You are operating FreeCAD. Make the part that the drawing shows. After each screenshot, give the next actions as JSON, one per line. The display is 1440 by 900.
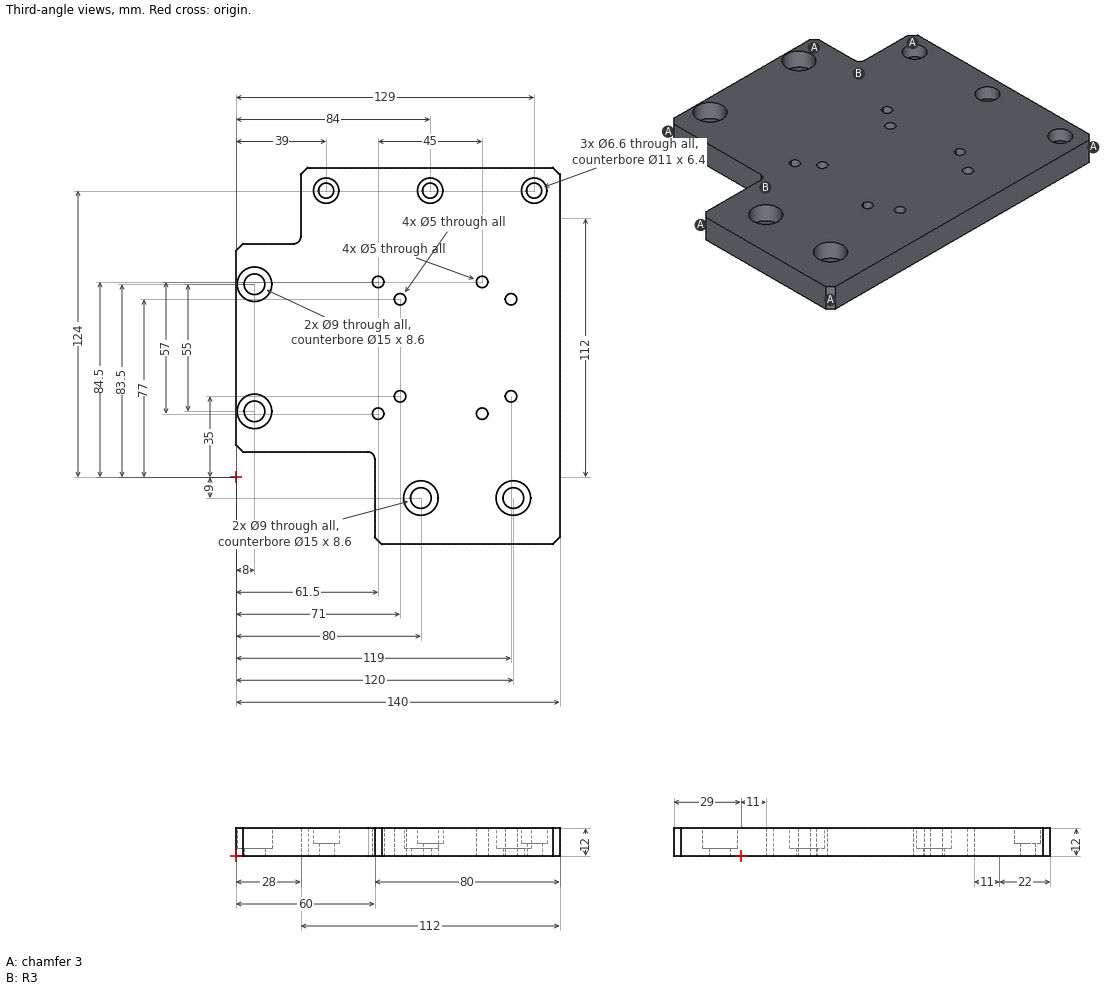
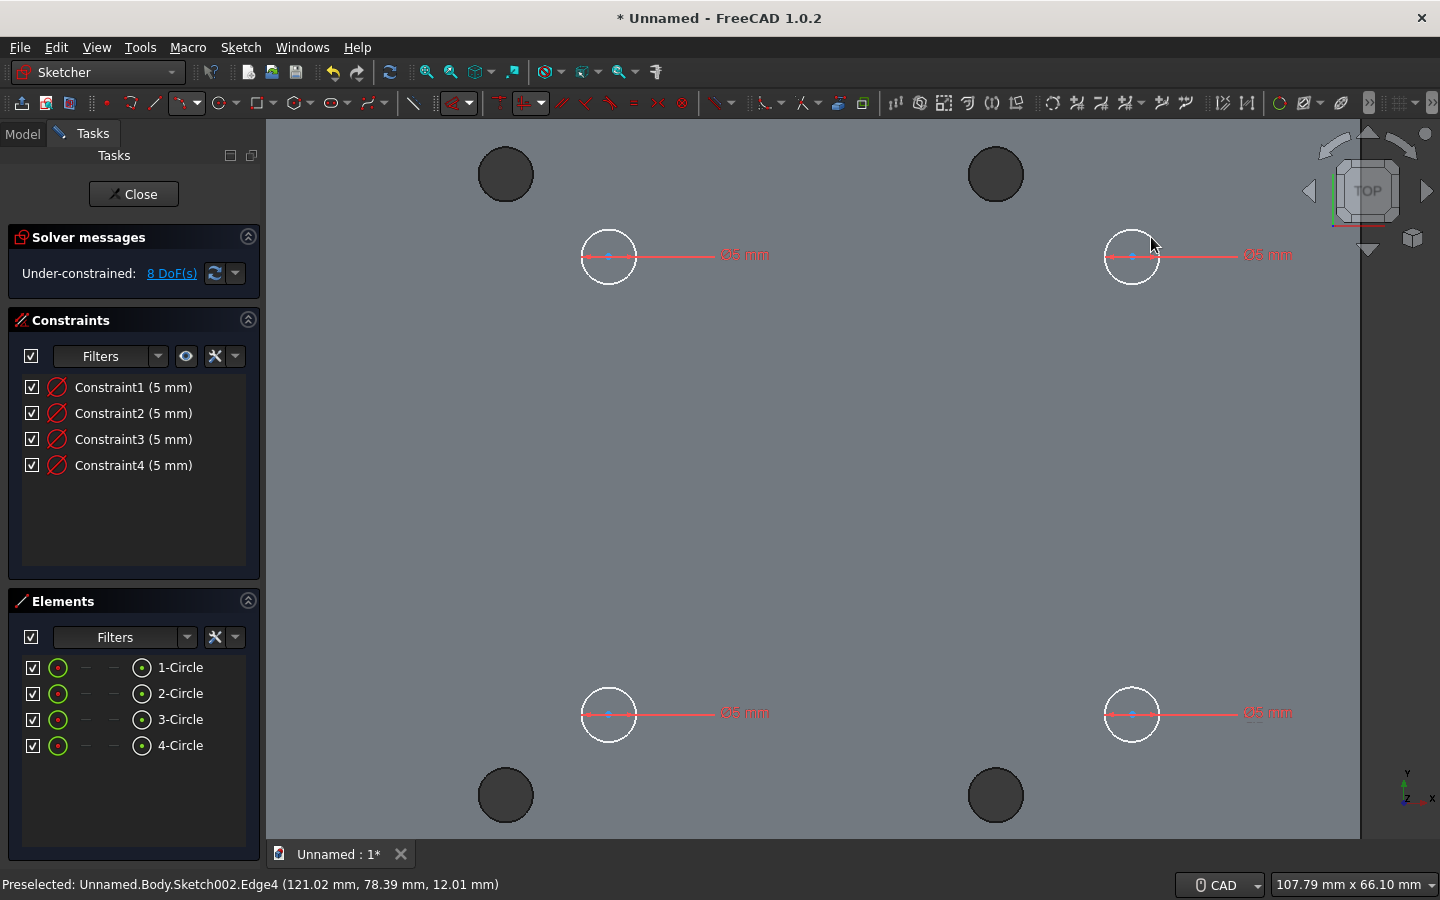
{"action": "left_click", "coordinate": [609, 257]}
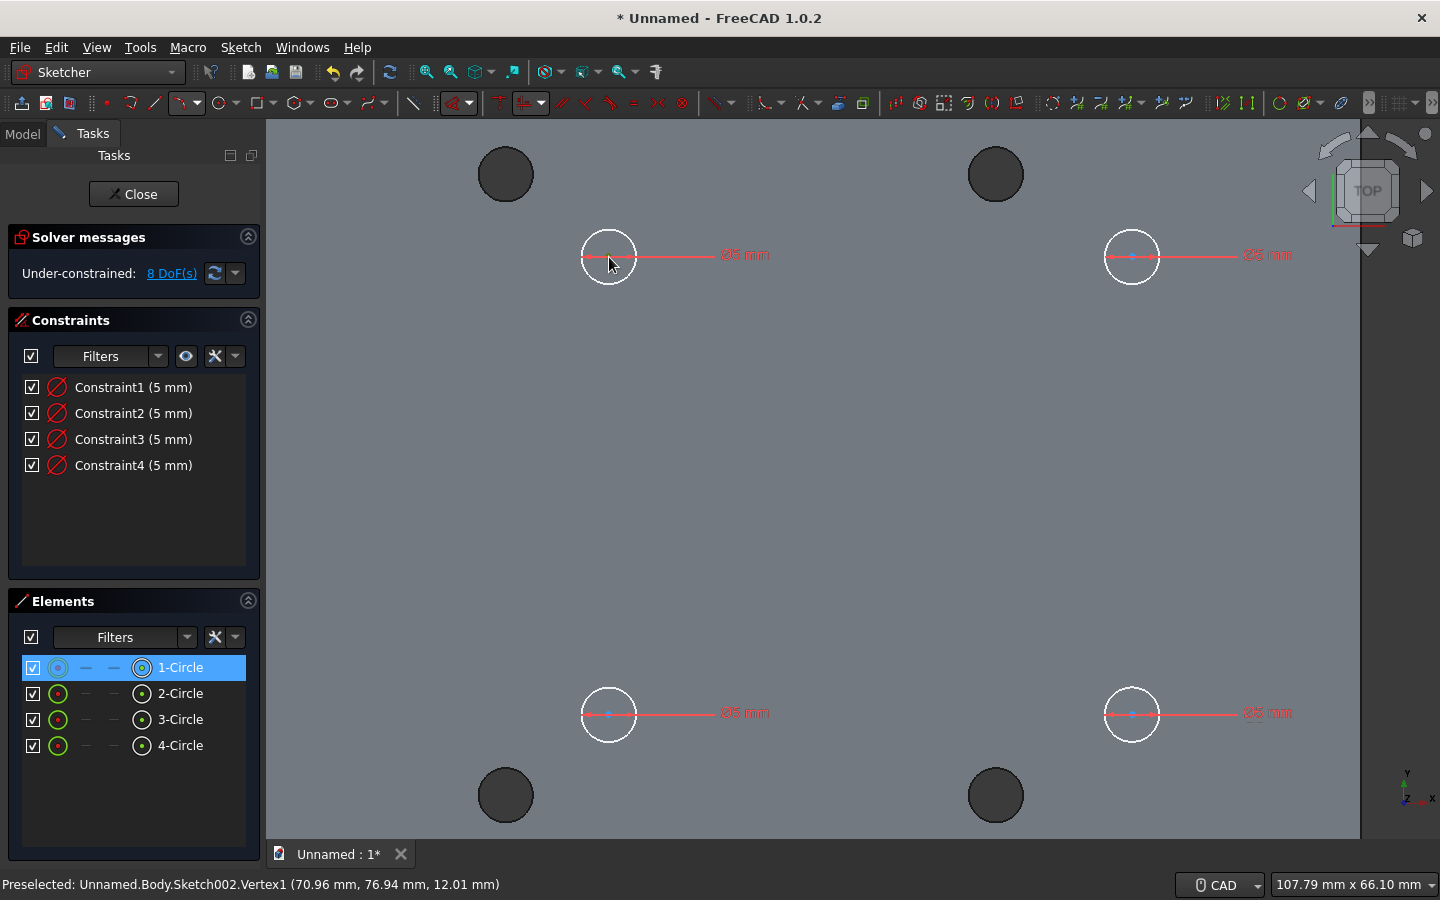
{"action": "key", "text": "l"}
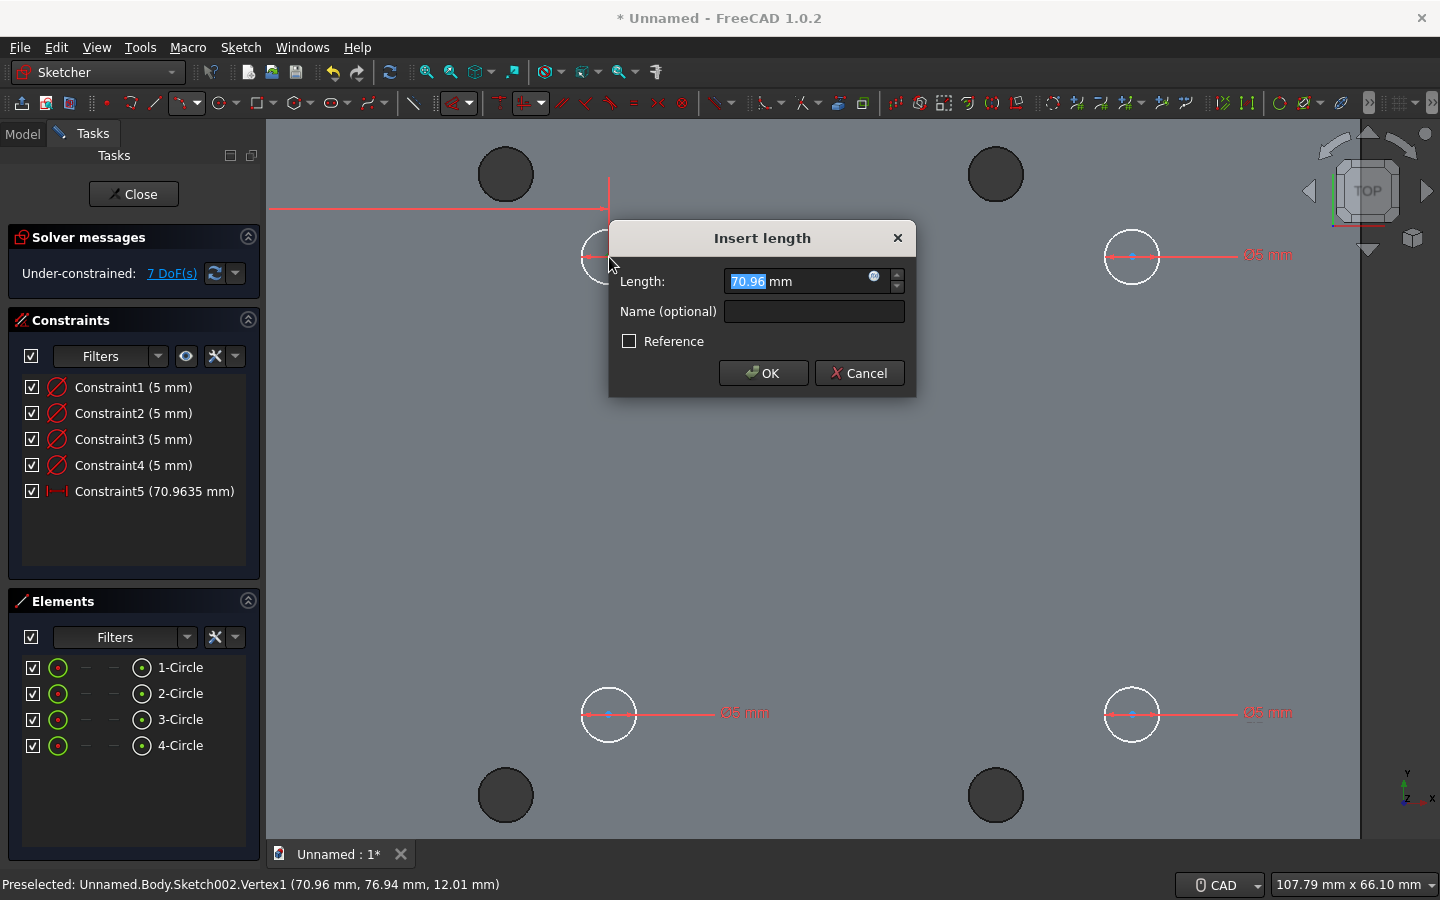
{"action": "type", "text": "71"}
{"action": "key", "text": "Return"}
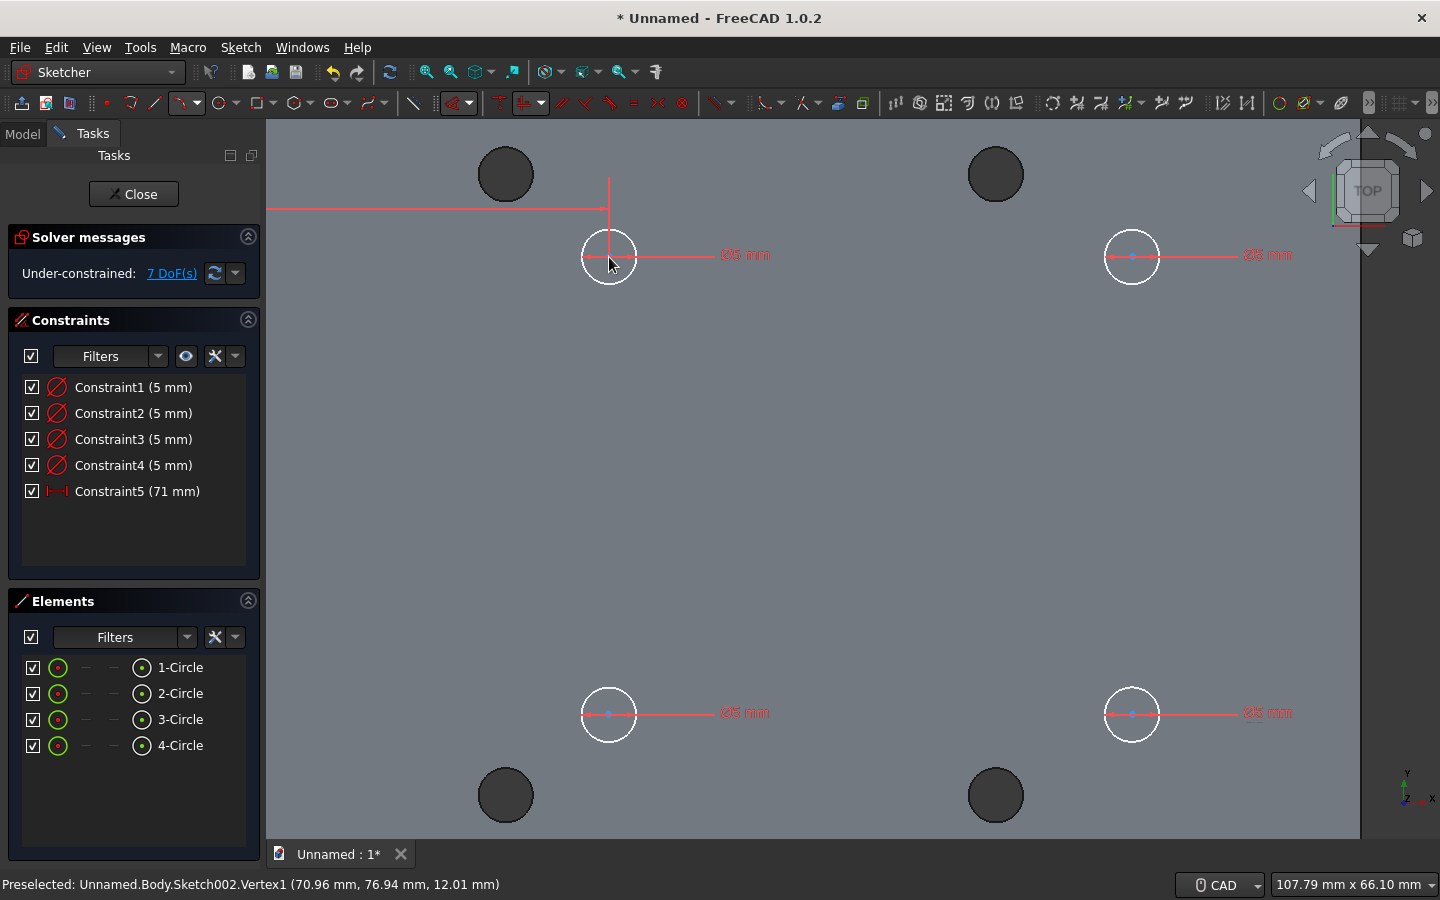
{"action": "left_click", "coordinate": [609, 257]}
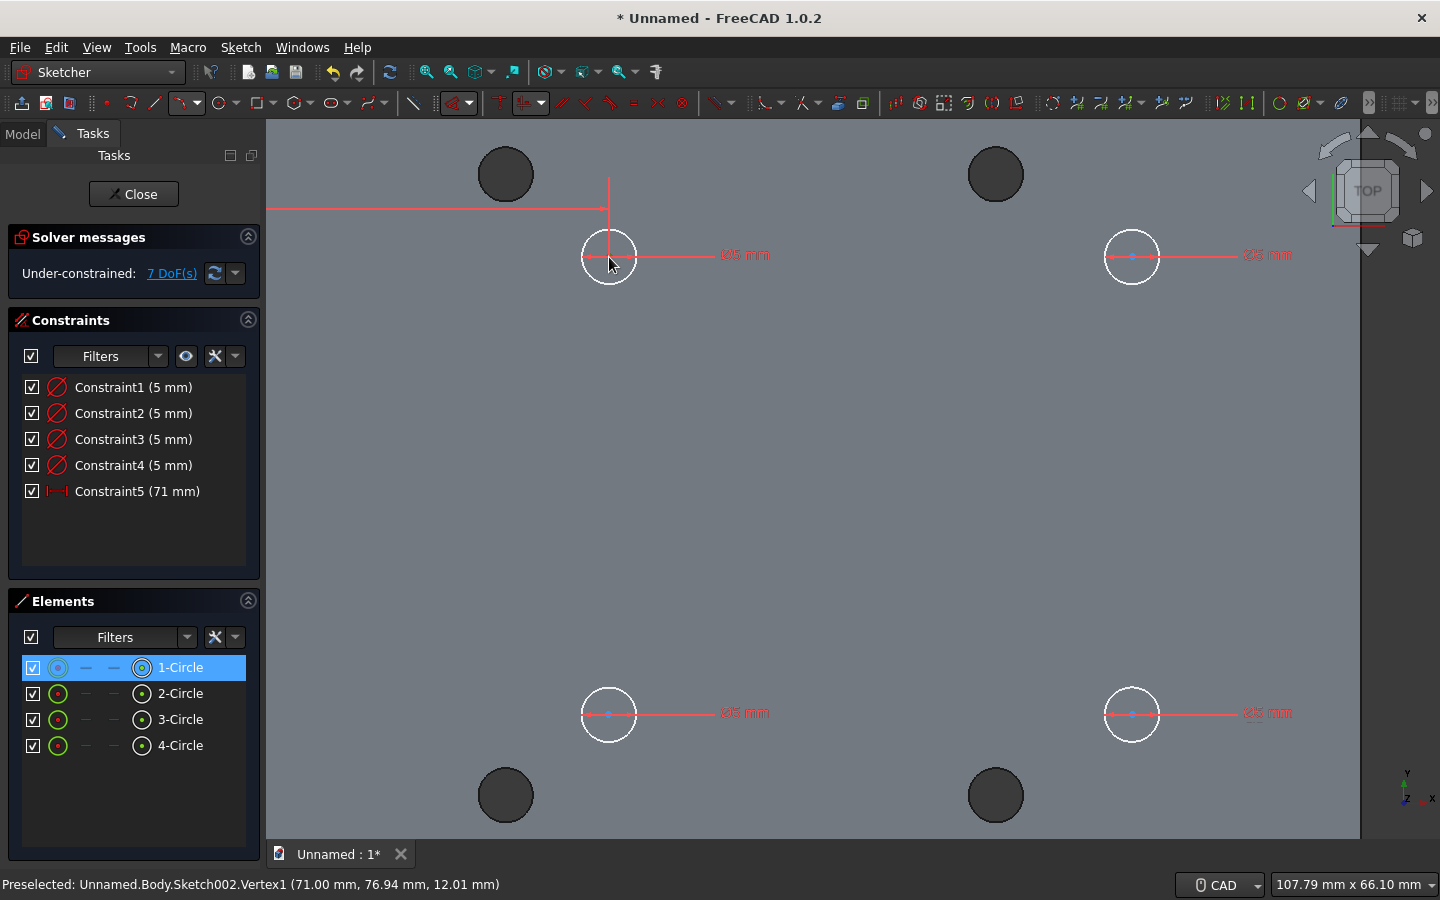
{"action": "key", "text": "i"}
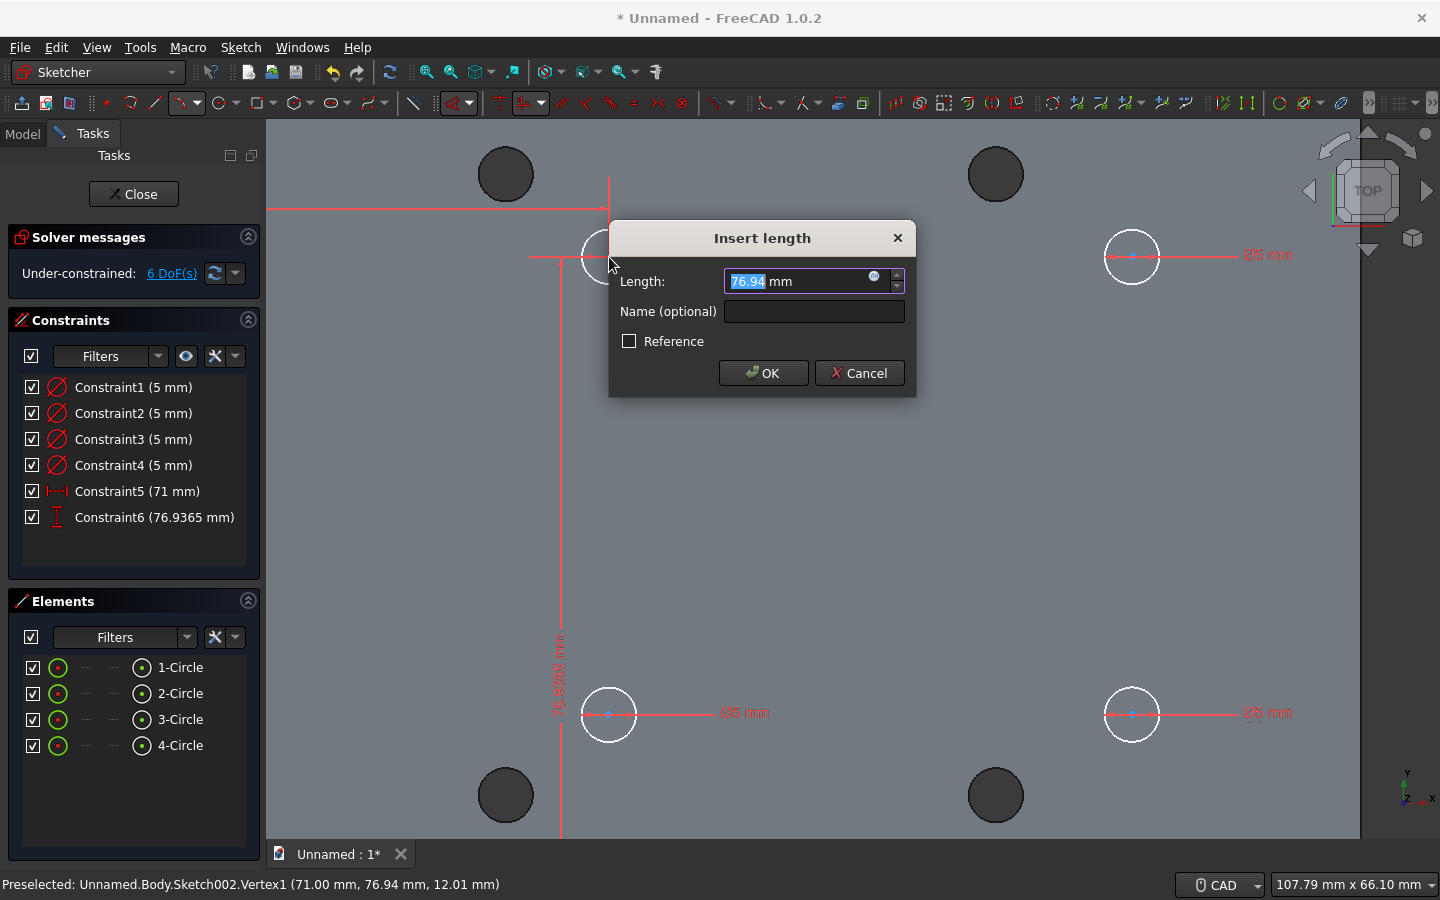
{"action": "type", "text": "77"}
{"action": "key", "text": "Return"}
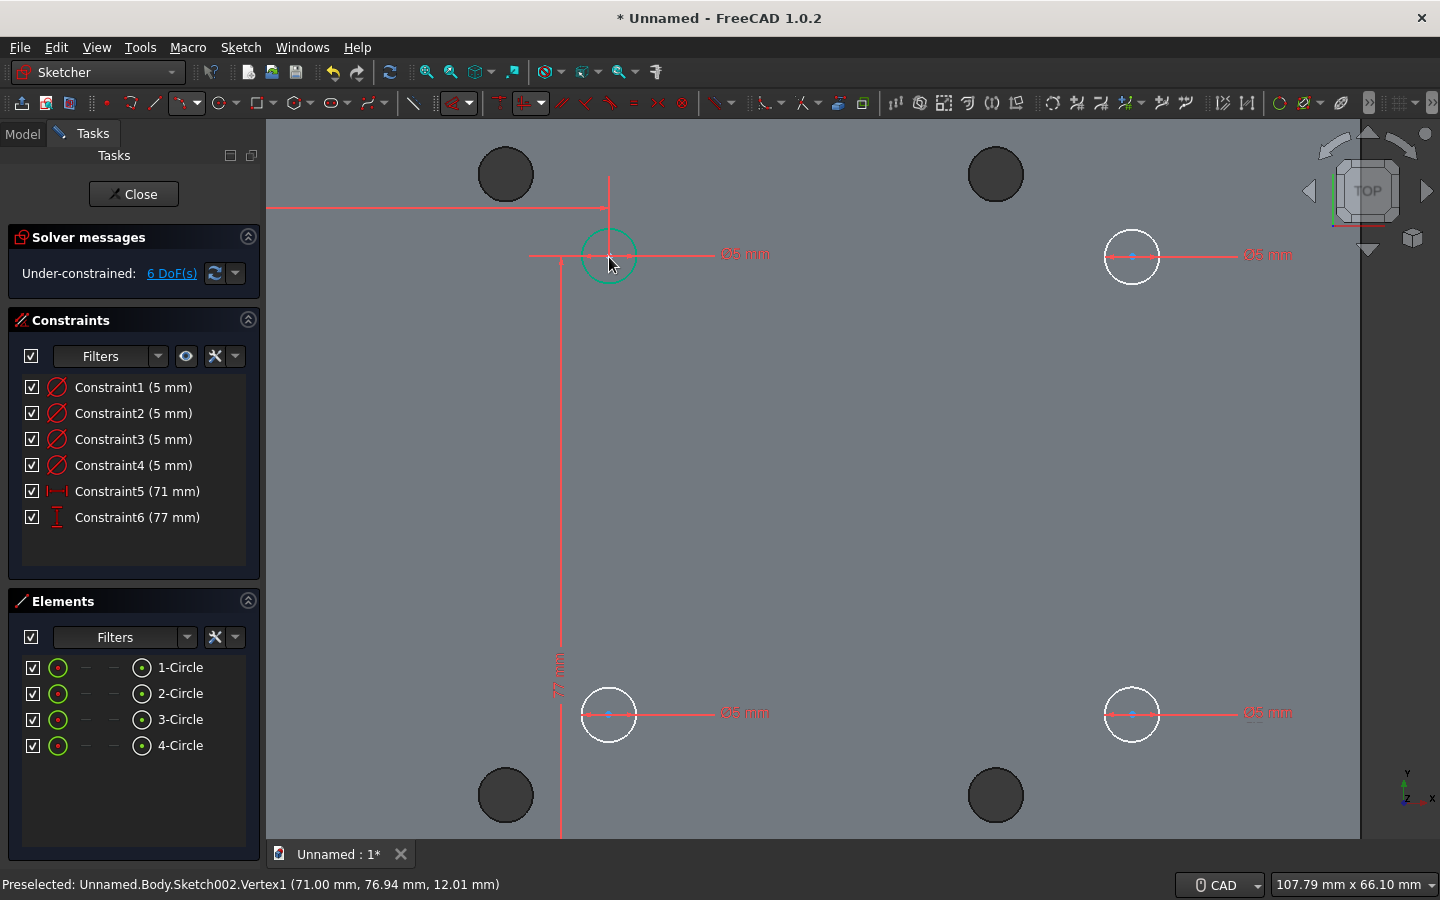
{"action": "left_click", "coordinate": [609, 715]}